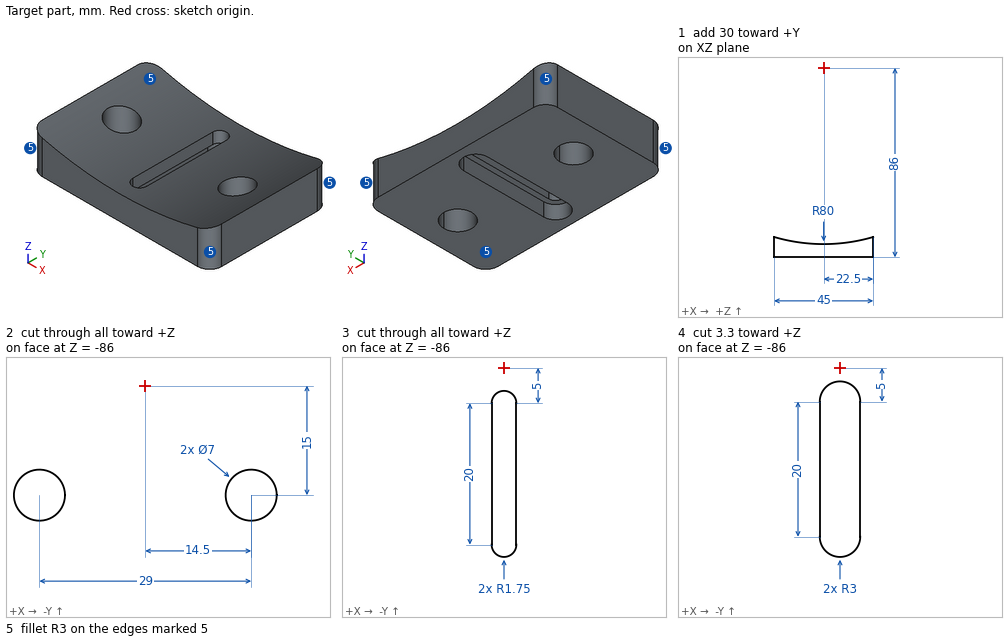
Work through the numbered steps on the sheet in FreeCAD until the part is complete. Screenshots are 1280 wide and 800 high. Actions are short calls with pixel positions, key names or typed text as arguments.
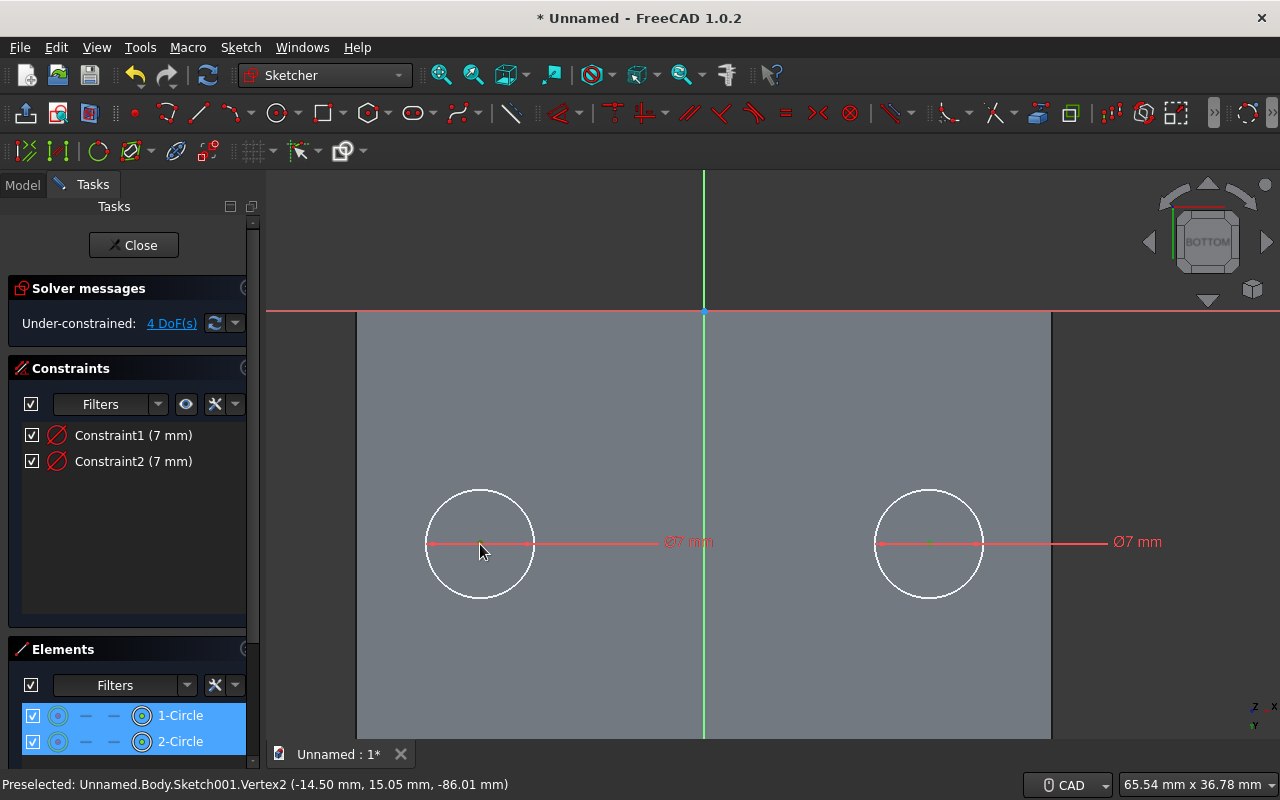
key(h)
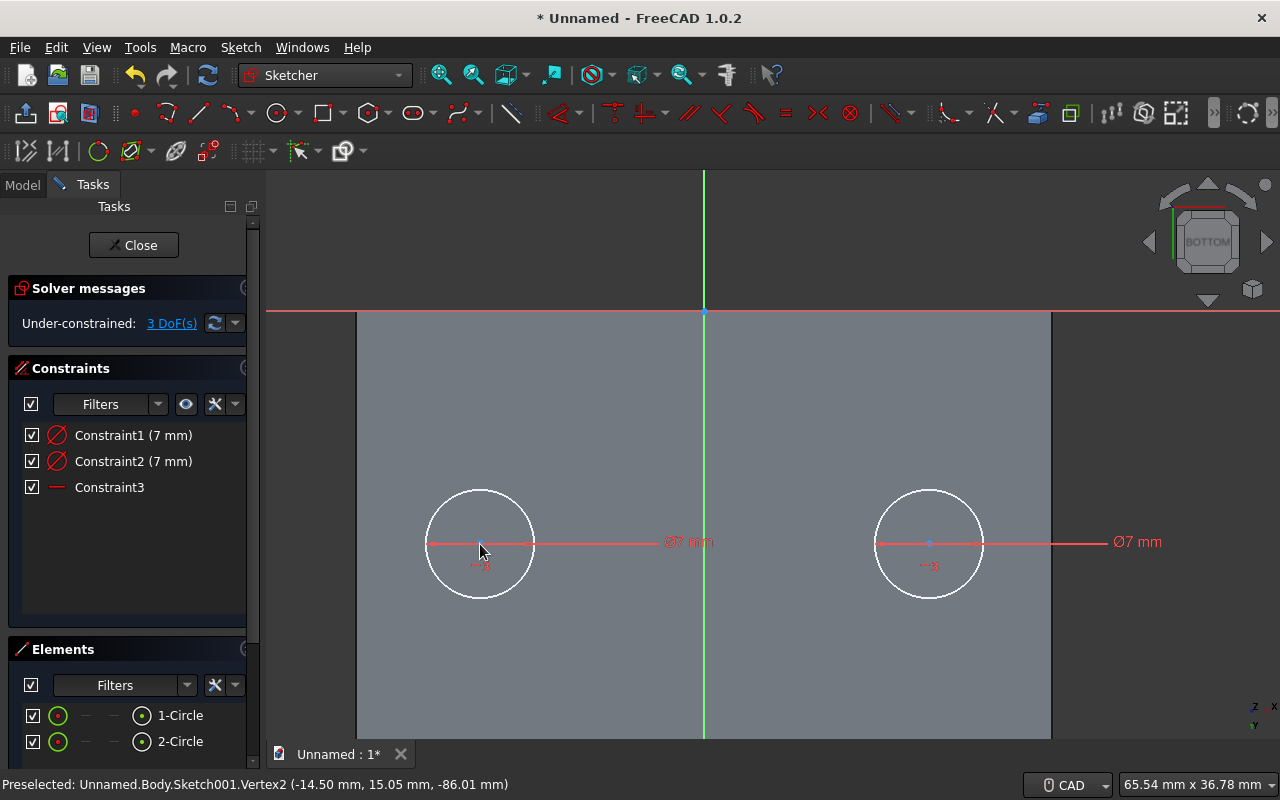
key(d)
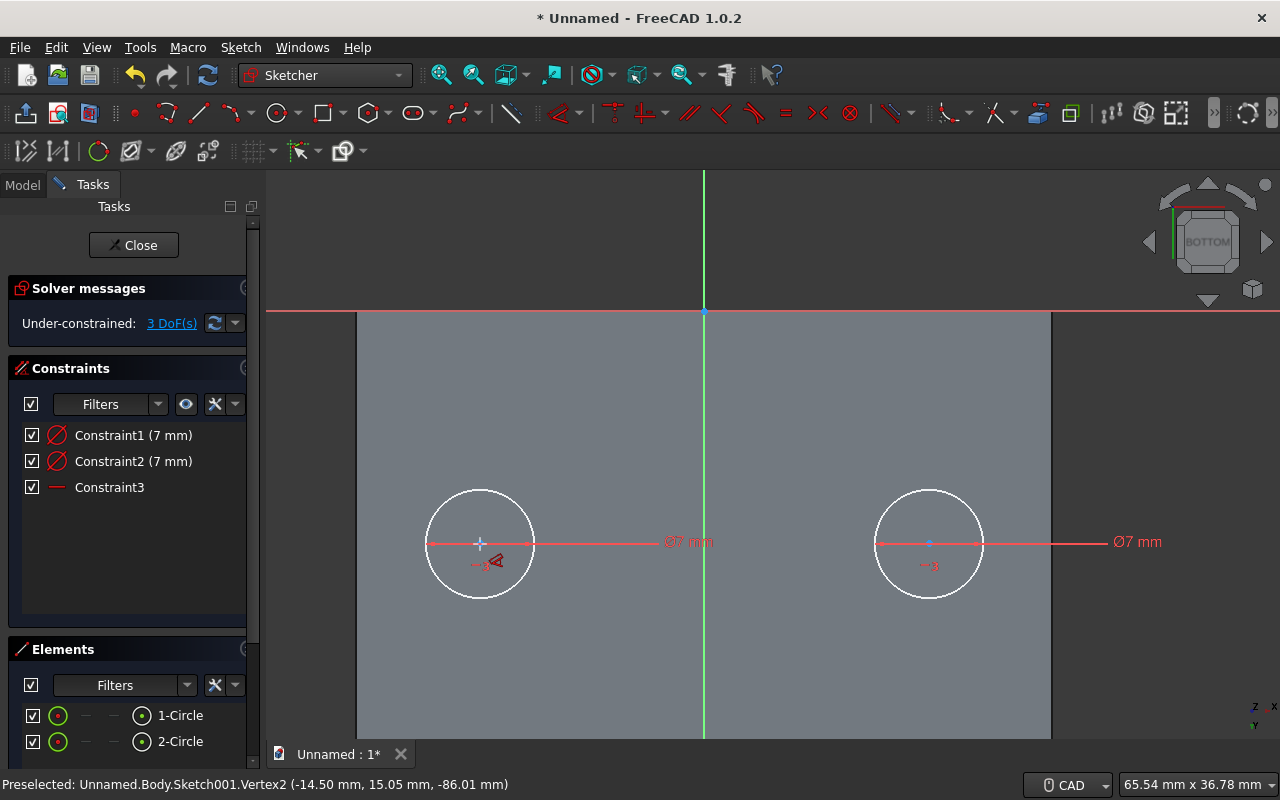
click(929, 544)
click(963, 428)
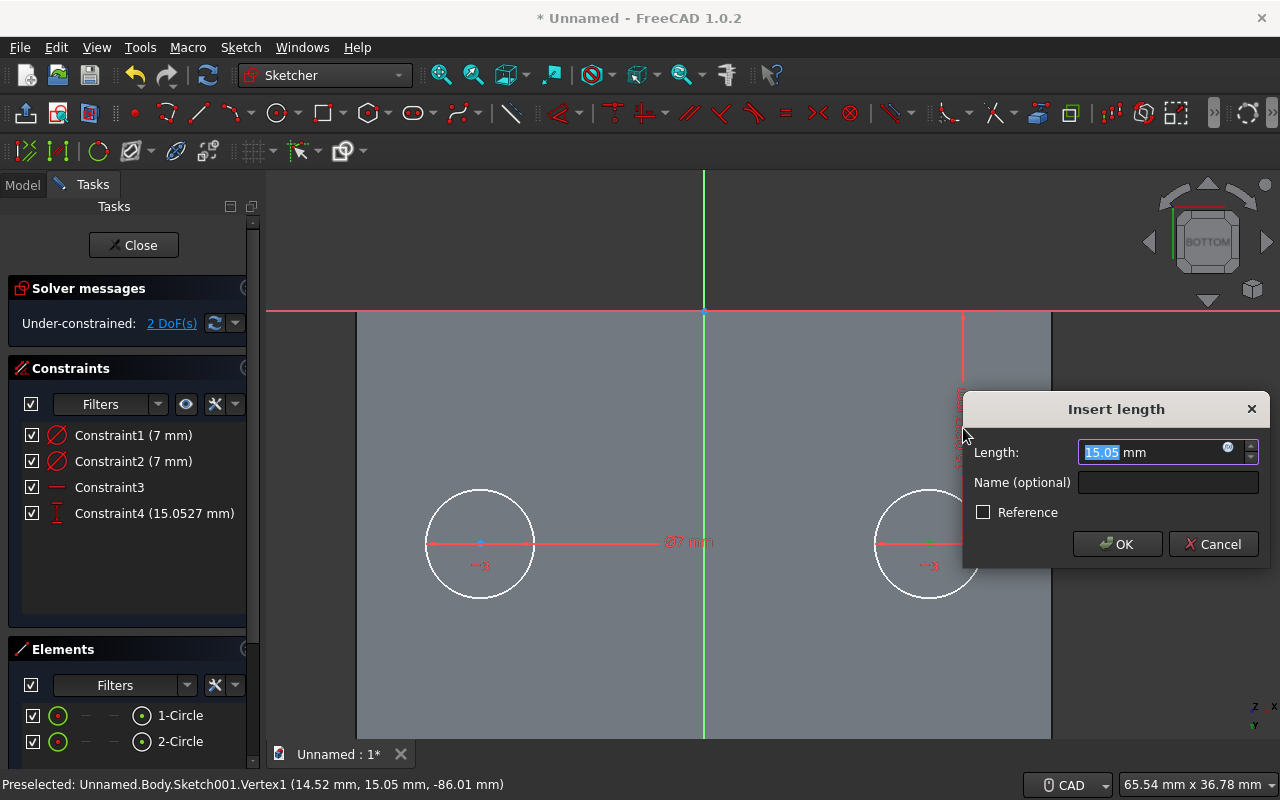
text(15)
key(Return)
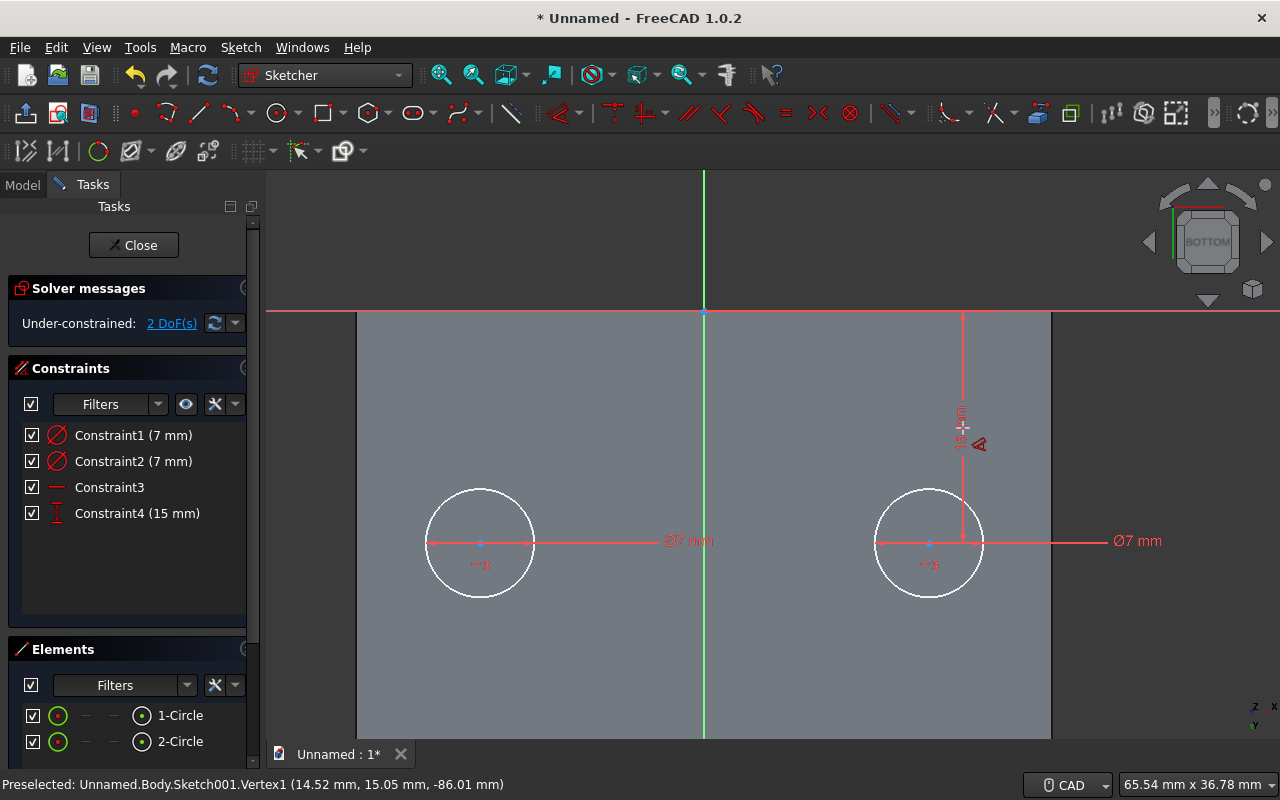
click(929, 543)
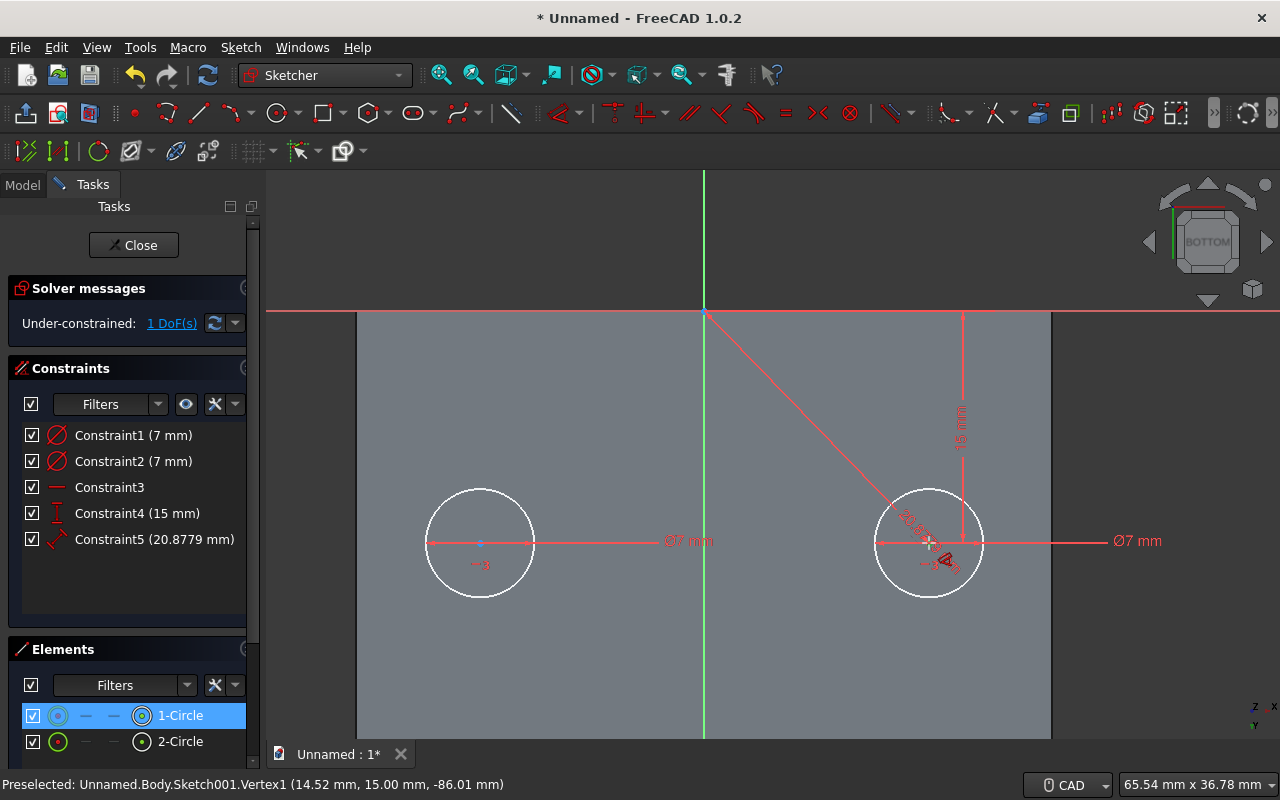
click(480, 543)
click(601, 577)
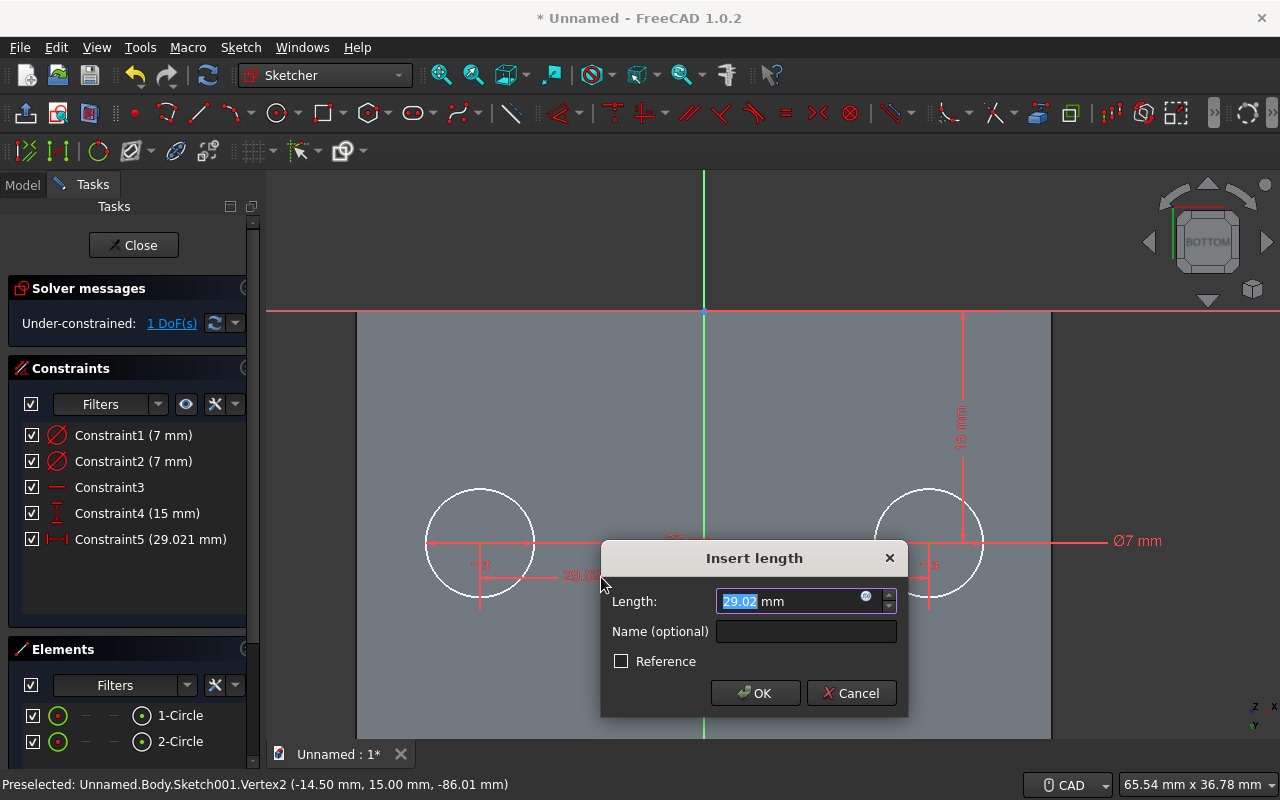
text(29)
key(Return)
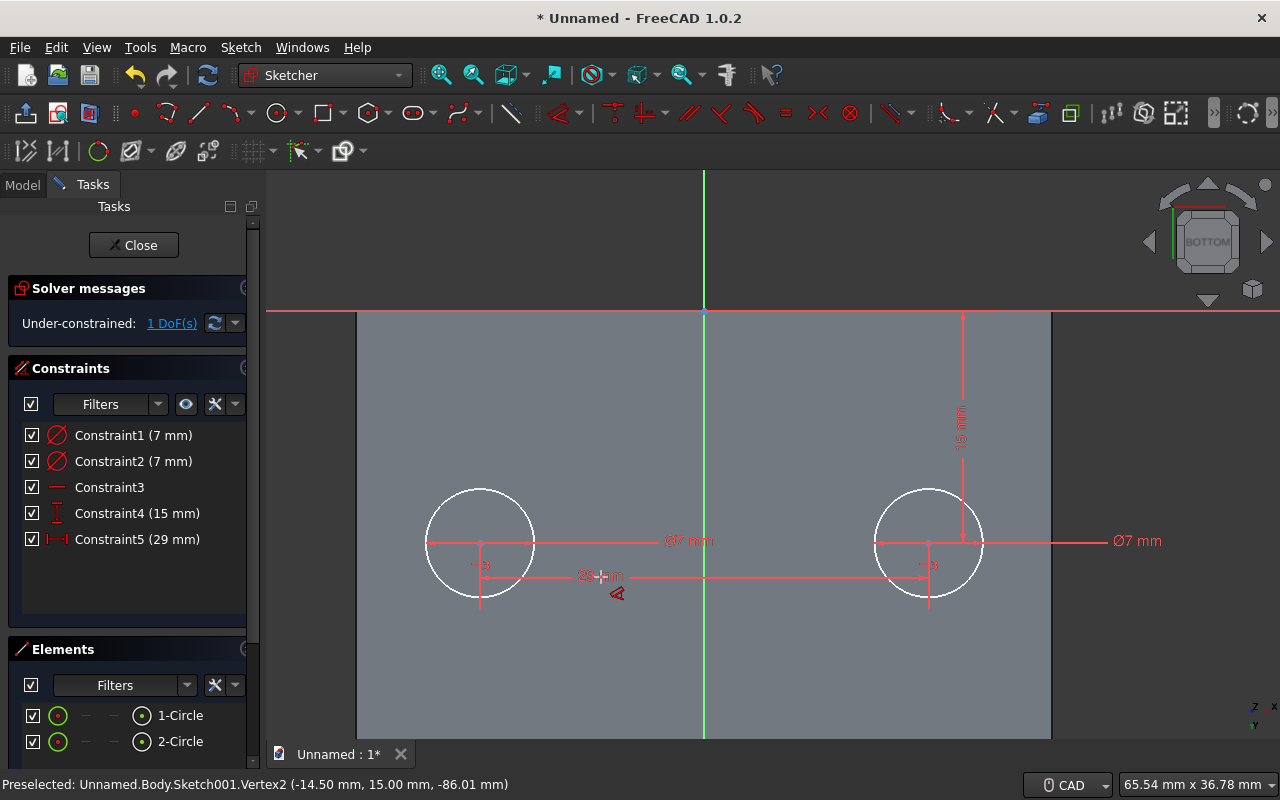
click(929, 543)
click(816, 277)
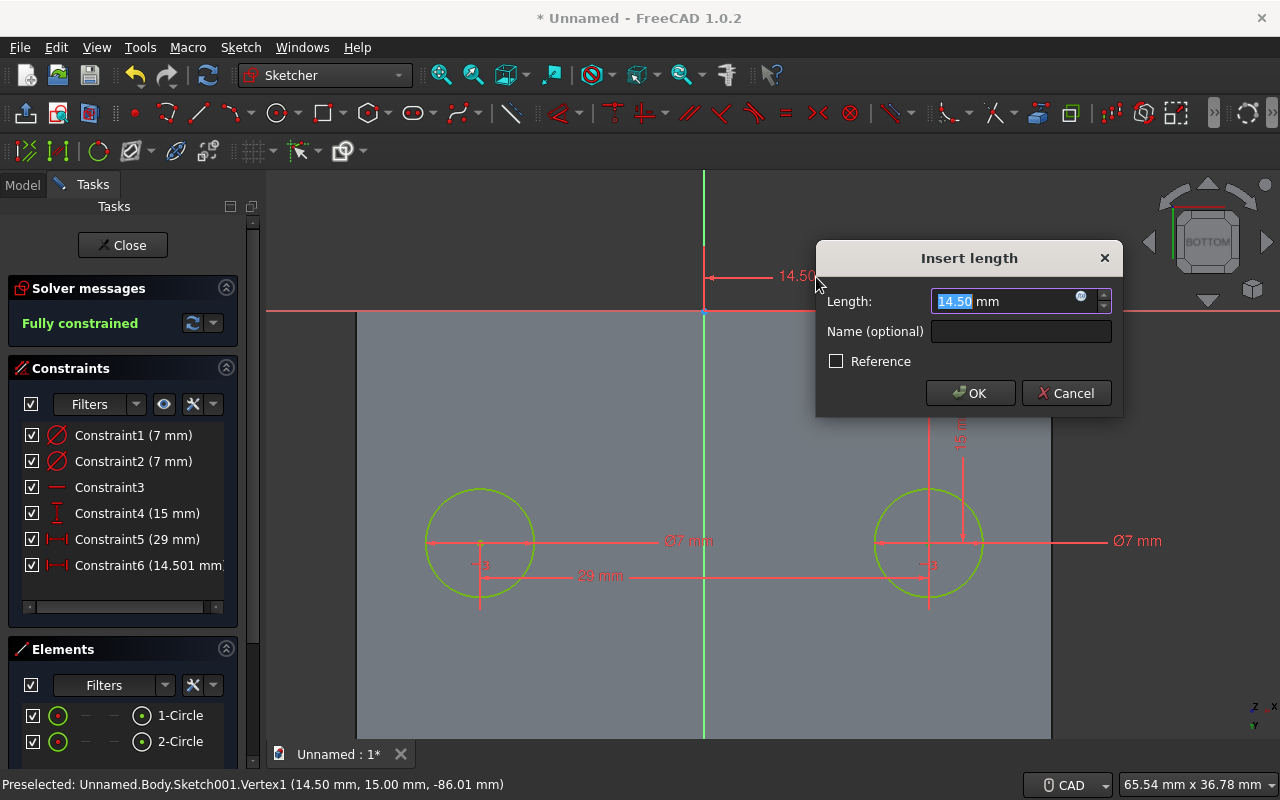
text(14.5)
key(Return)
key(Escape)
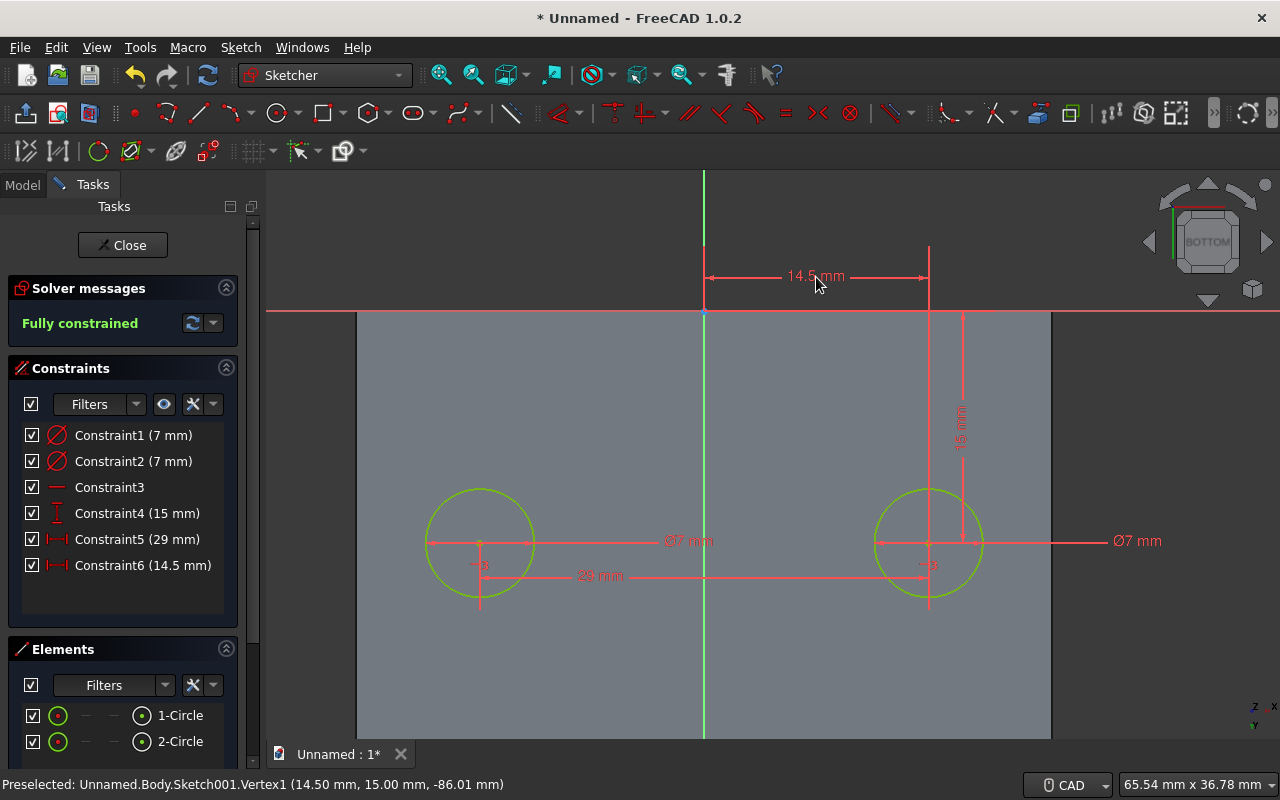
click(123, 245)